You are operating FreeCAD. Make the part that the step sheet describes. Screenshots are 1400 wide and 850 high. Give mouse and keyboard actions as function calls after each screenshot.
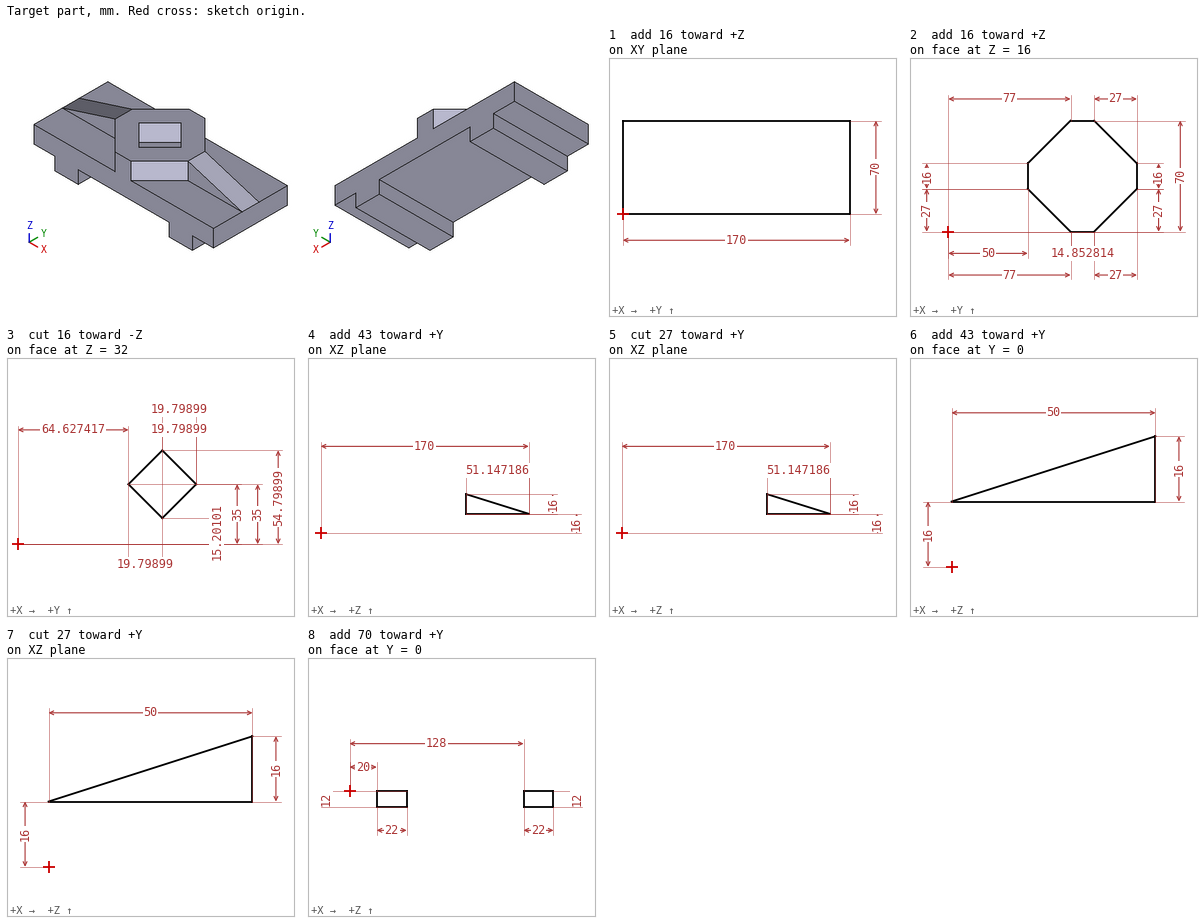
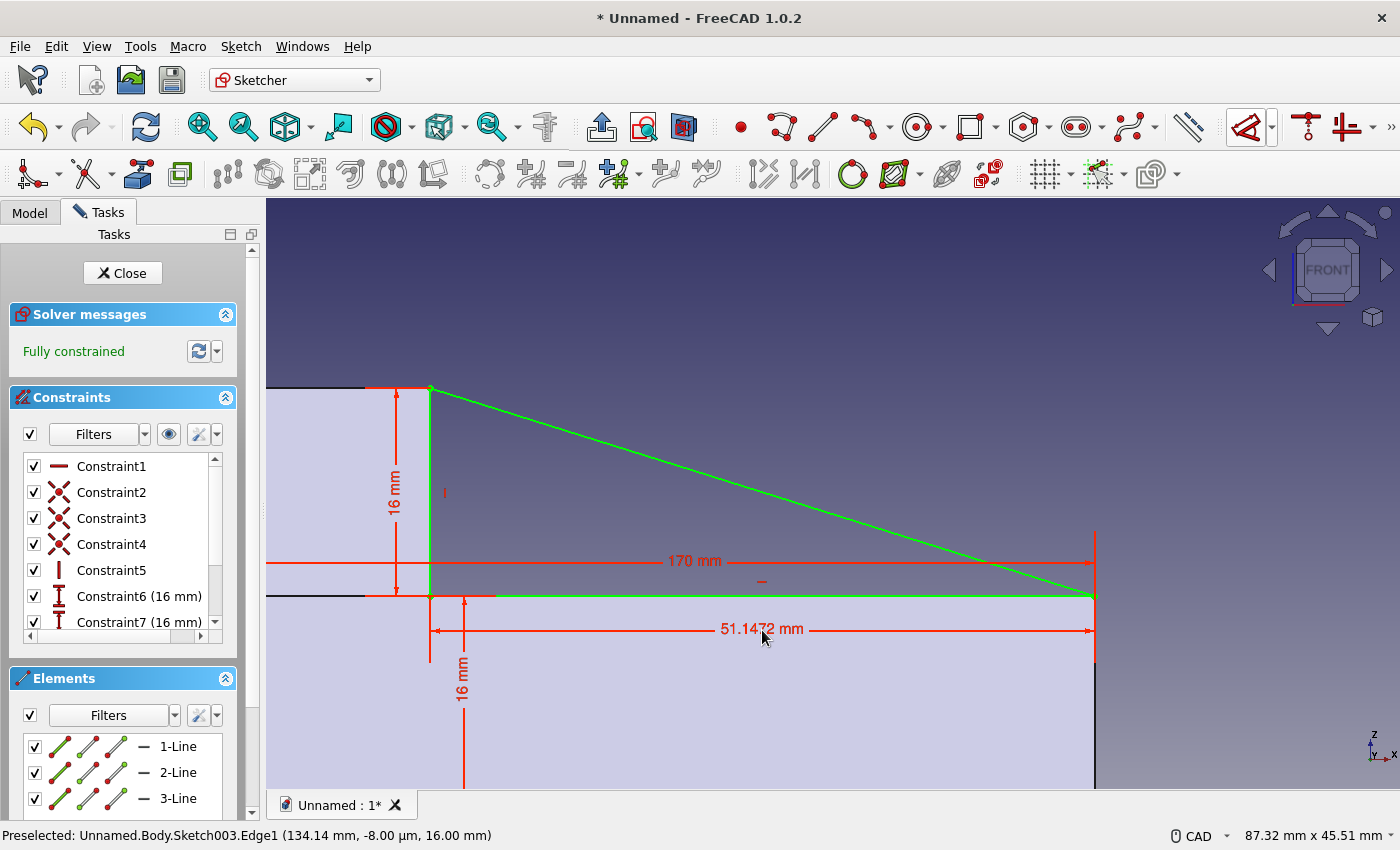
click(123, 273)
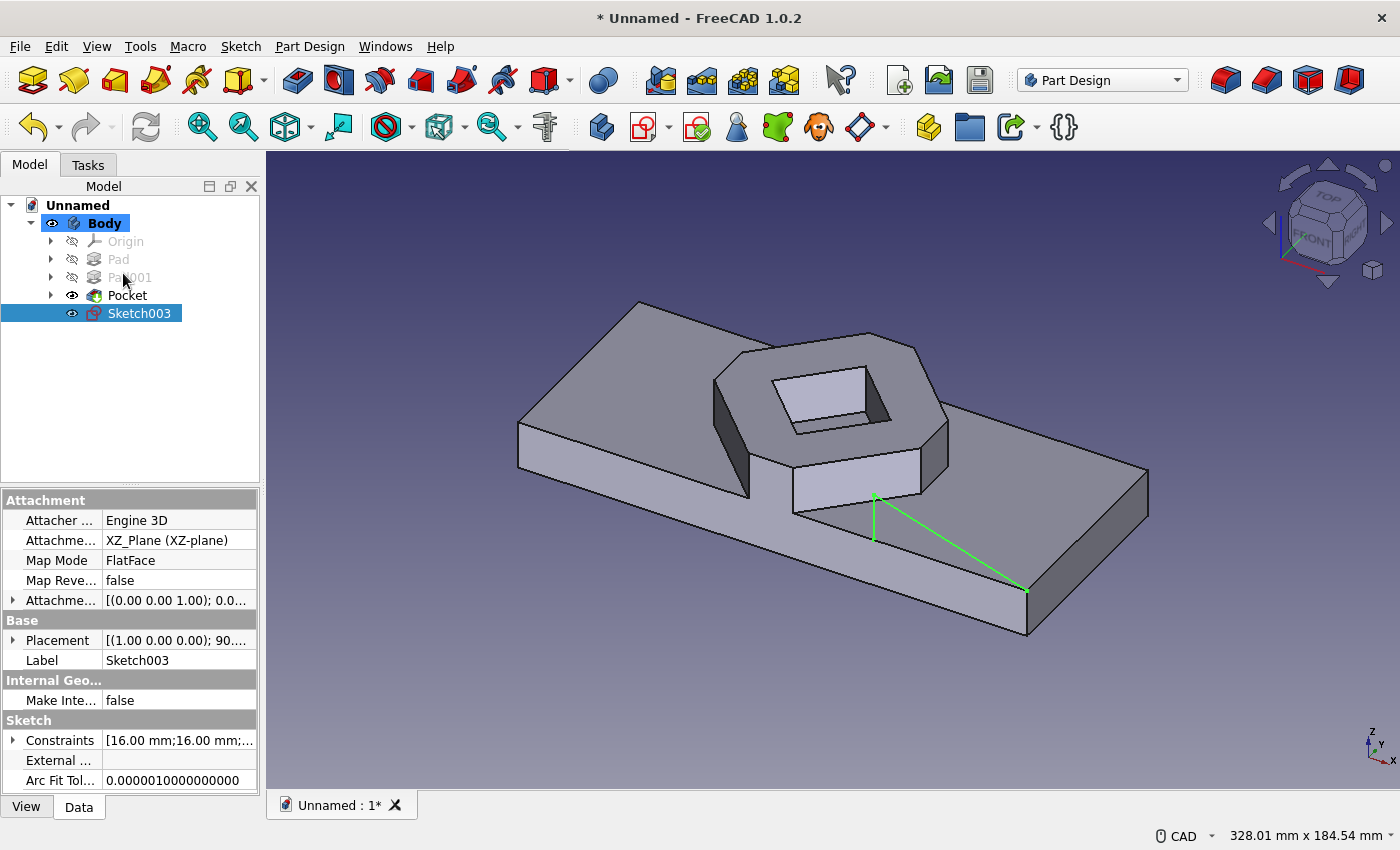
click(33, 80)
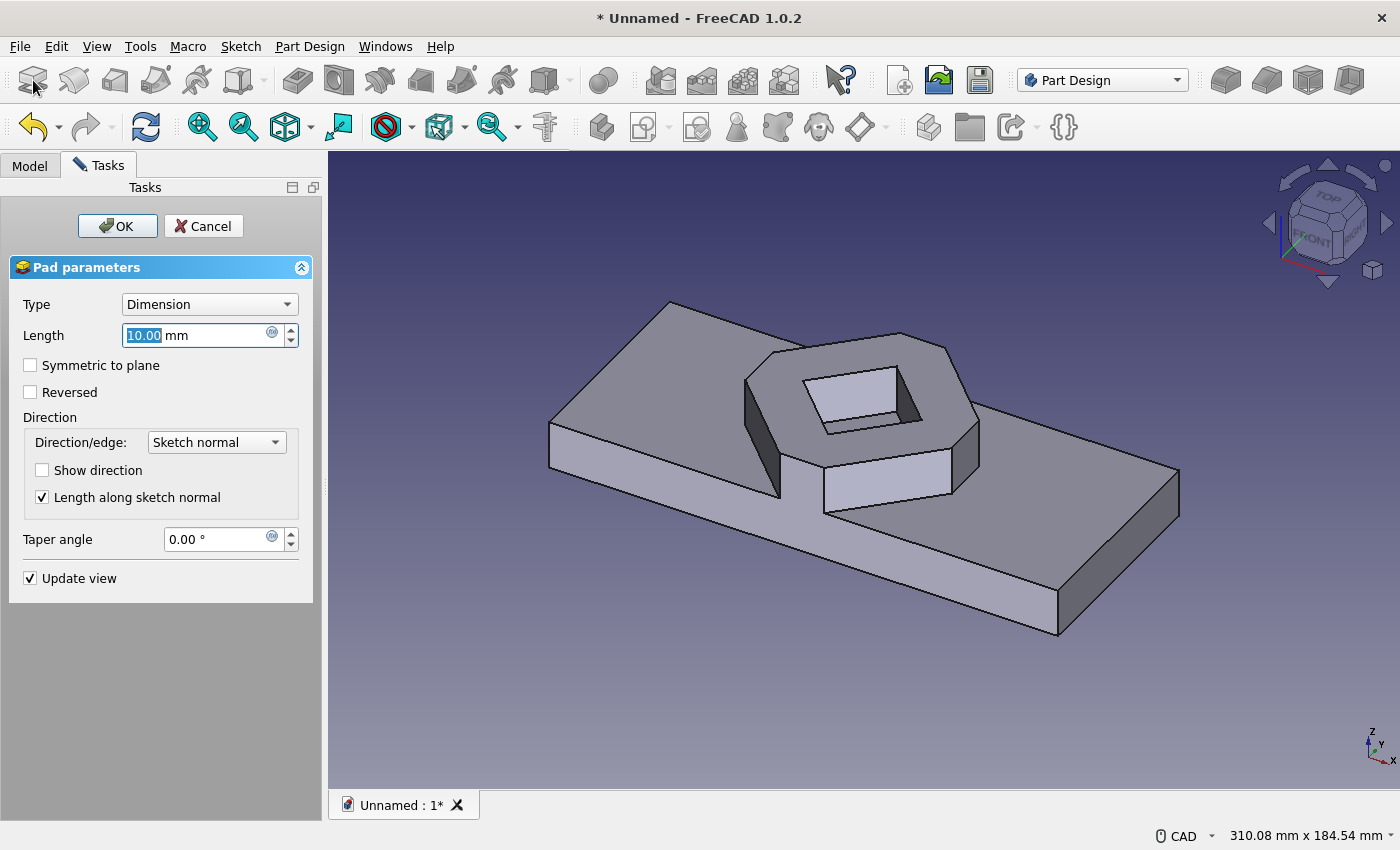
text(43)
key(Tab)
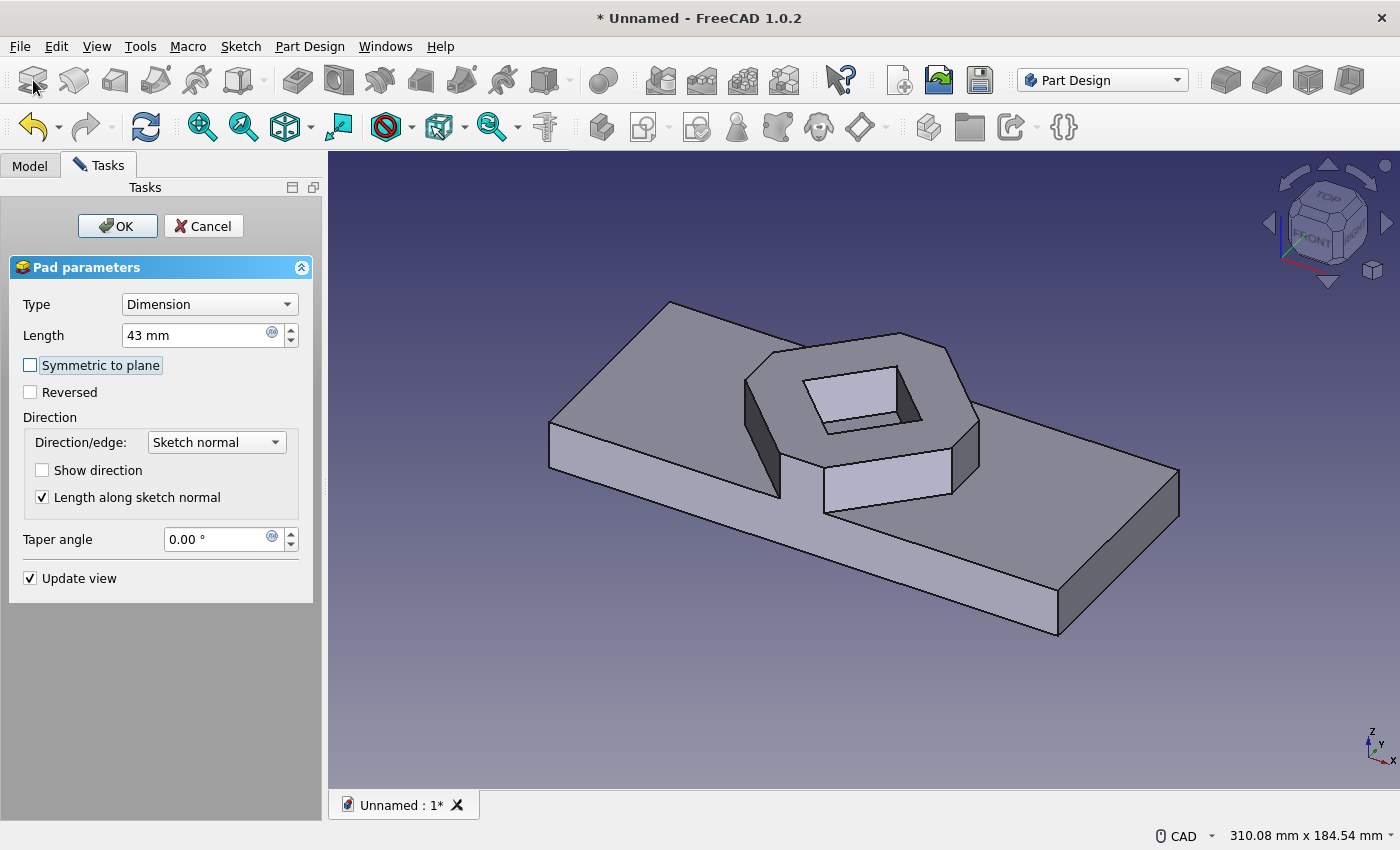
click(31, 392)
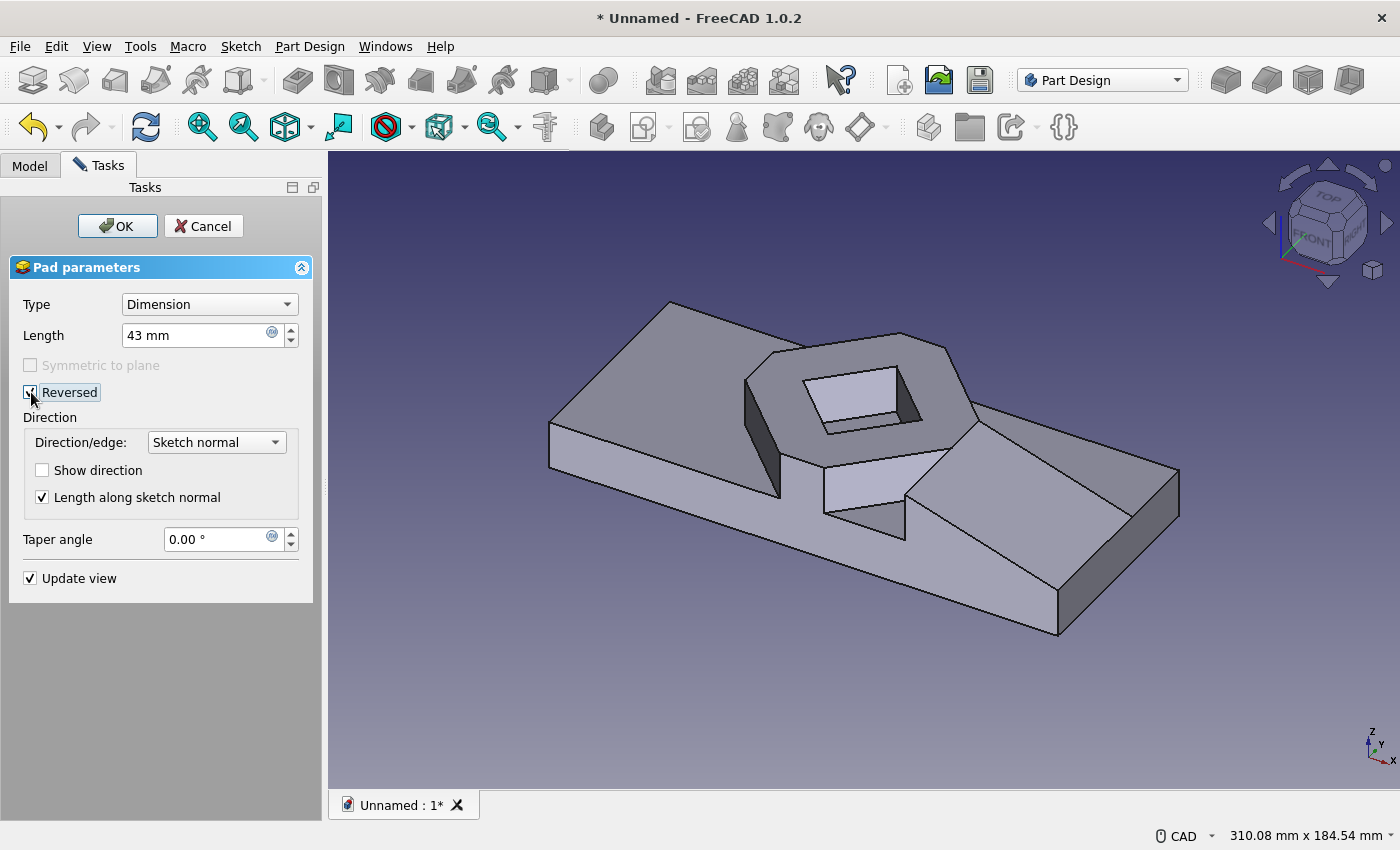
click(118, 226)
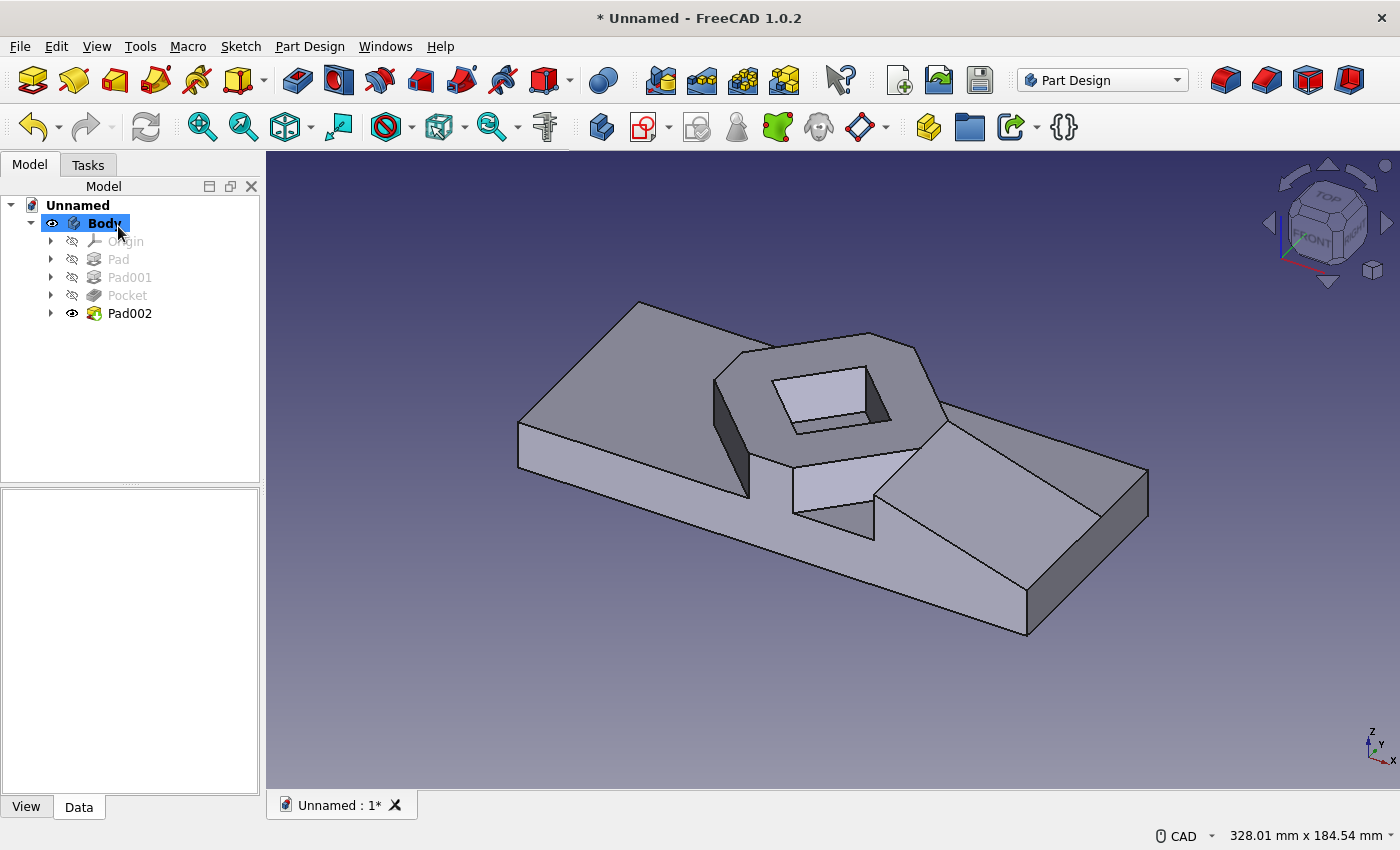
click(642, 128)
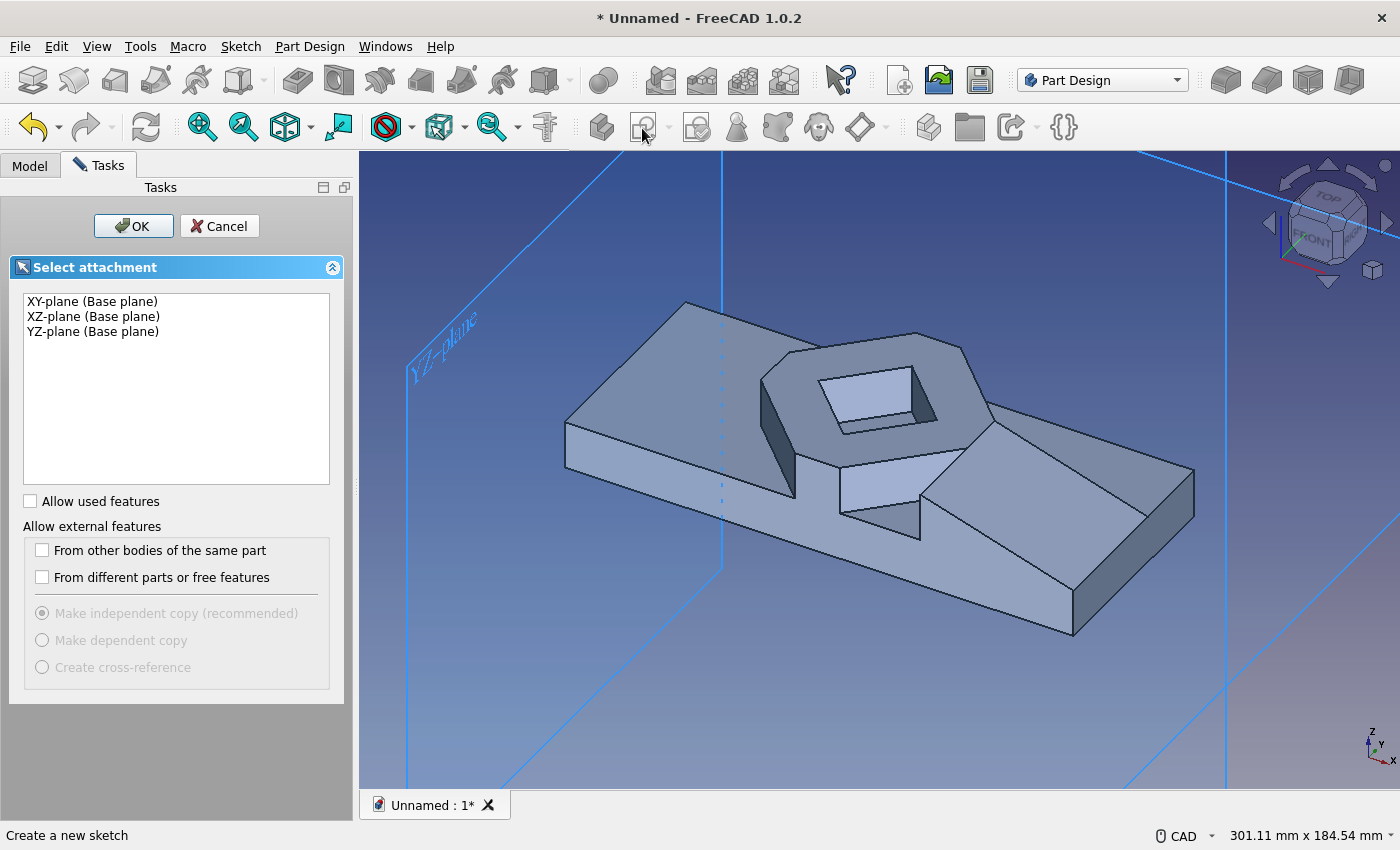
click(84, 316)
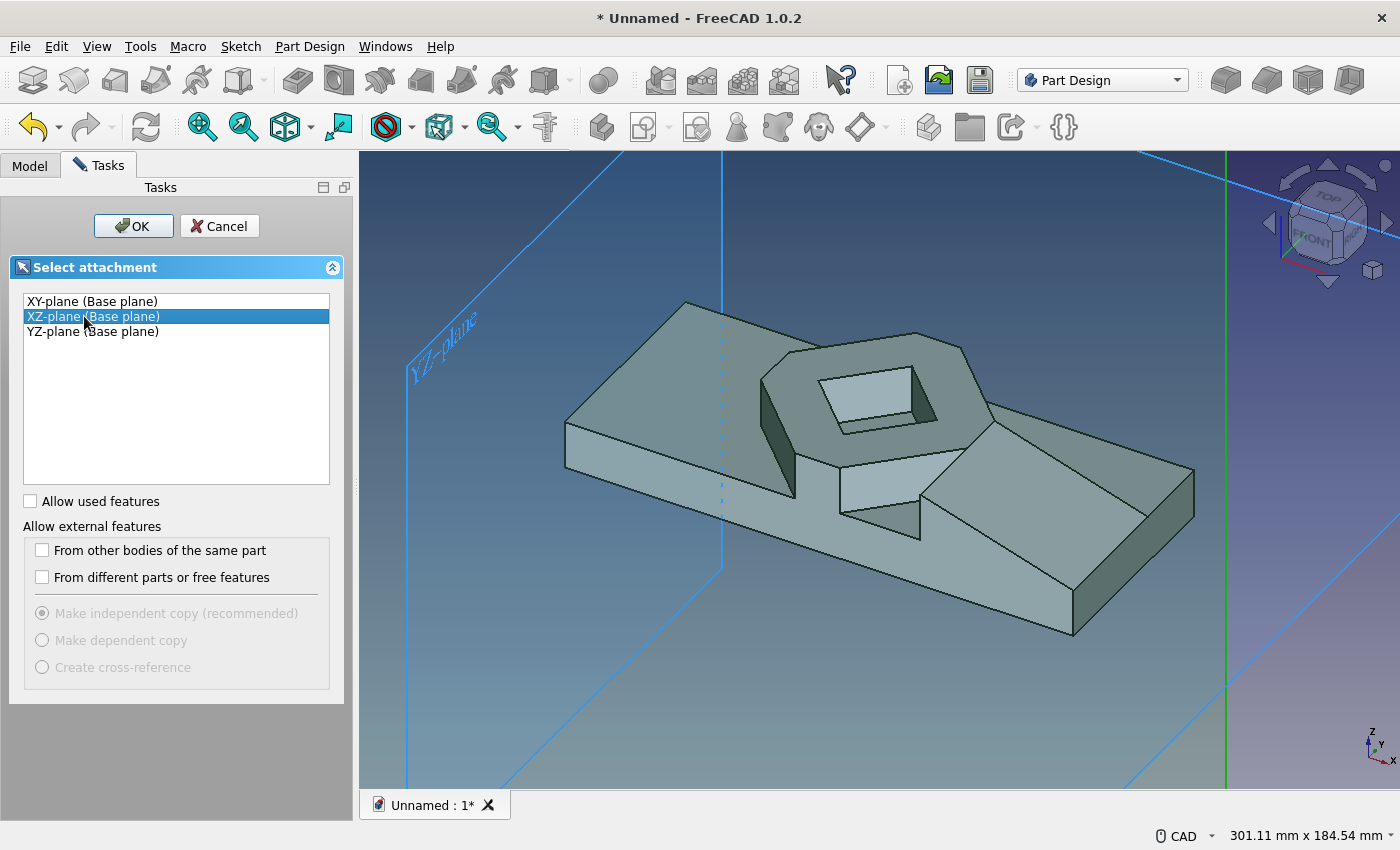
click(134, 226)